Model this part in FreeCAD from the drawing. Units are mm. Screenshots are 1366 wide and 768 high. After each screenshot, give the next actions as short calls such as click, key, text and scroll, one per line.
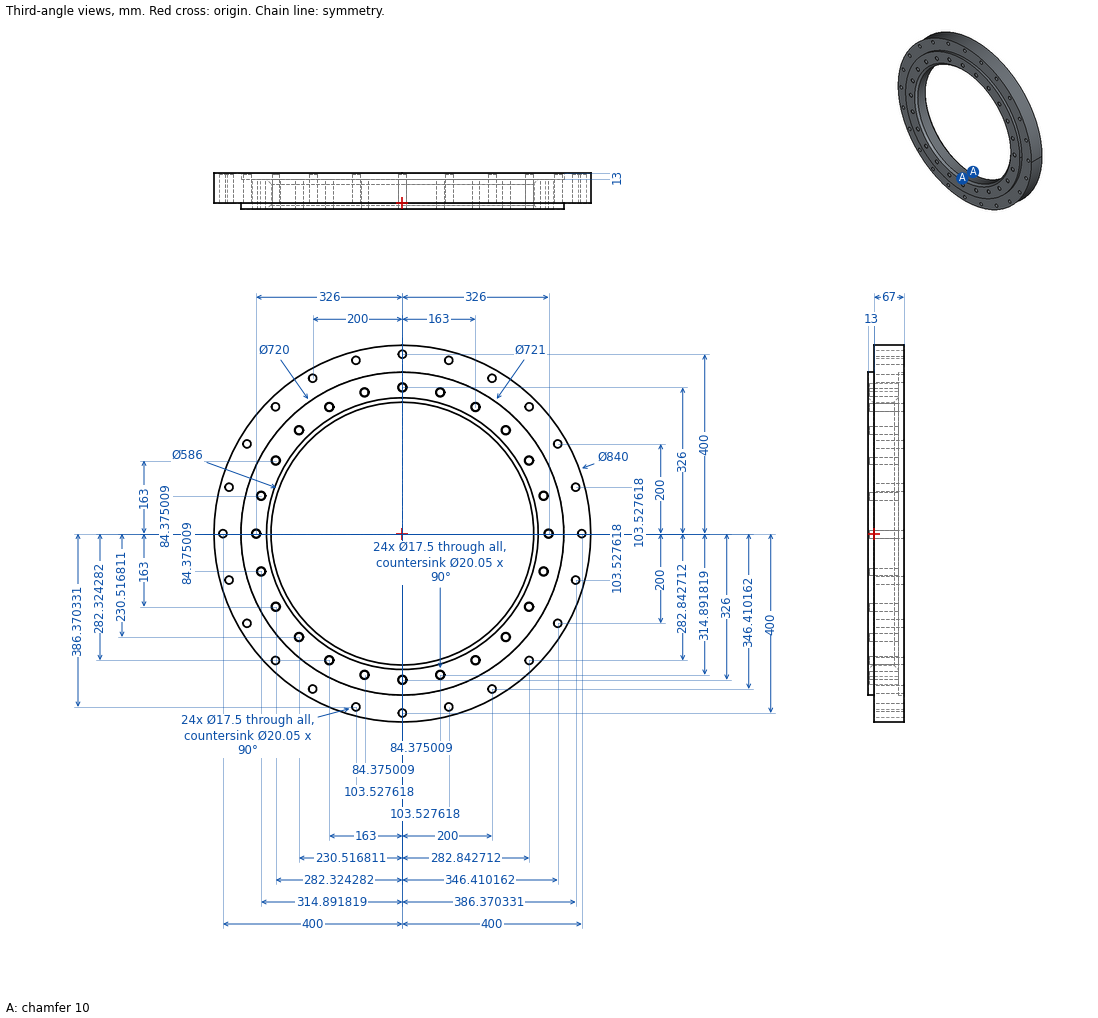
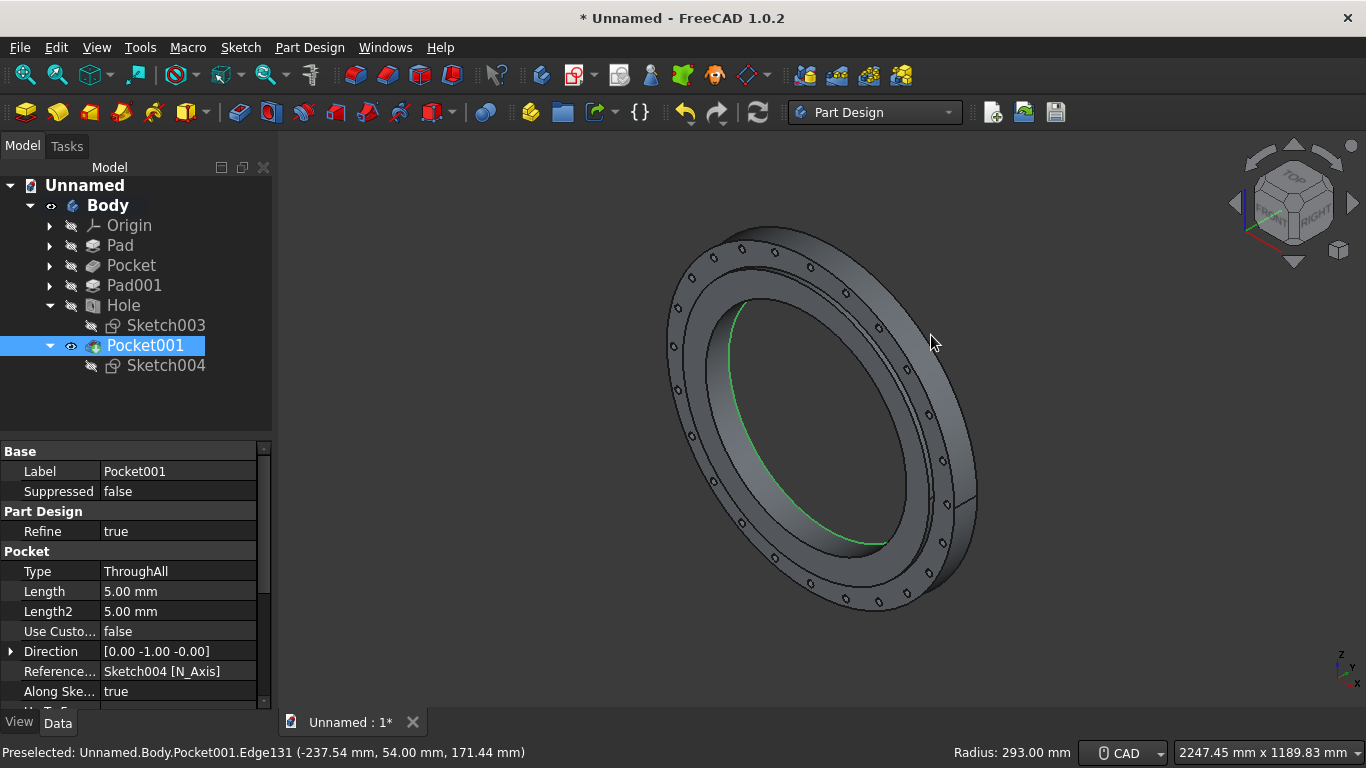
click(706, 369, ctrl)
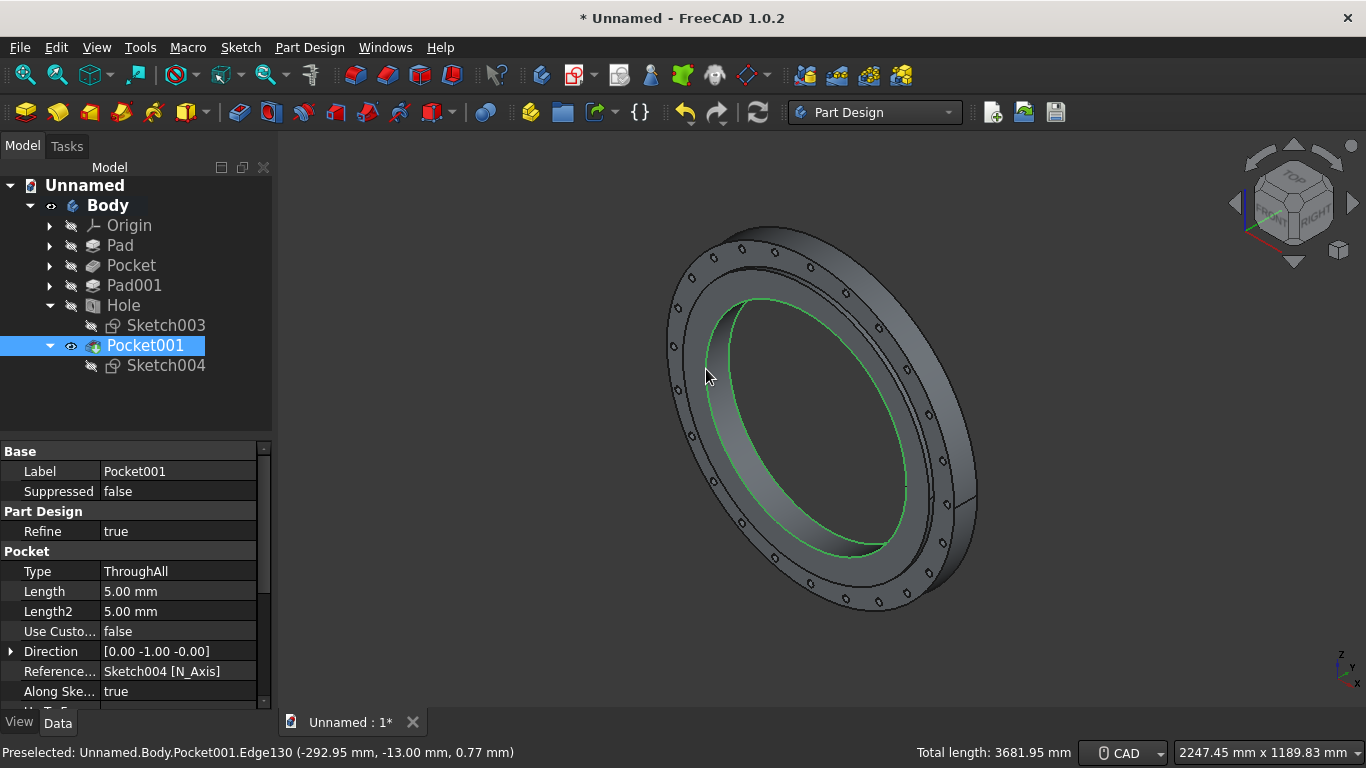
click(388, 76)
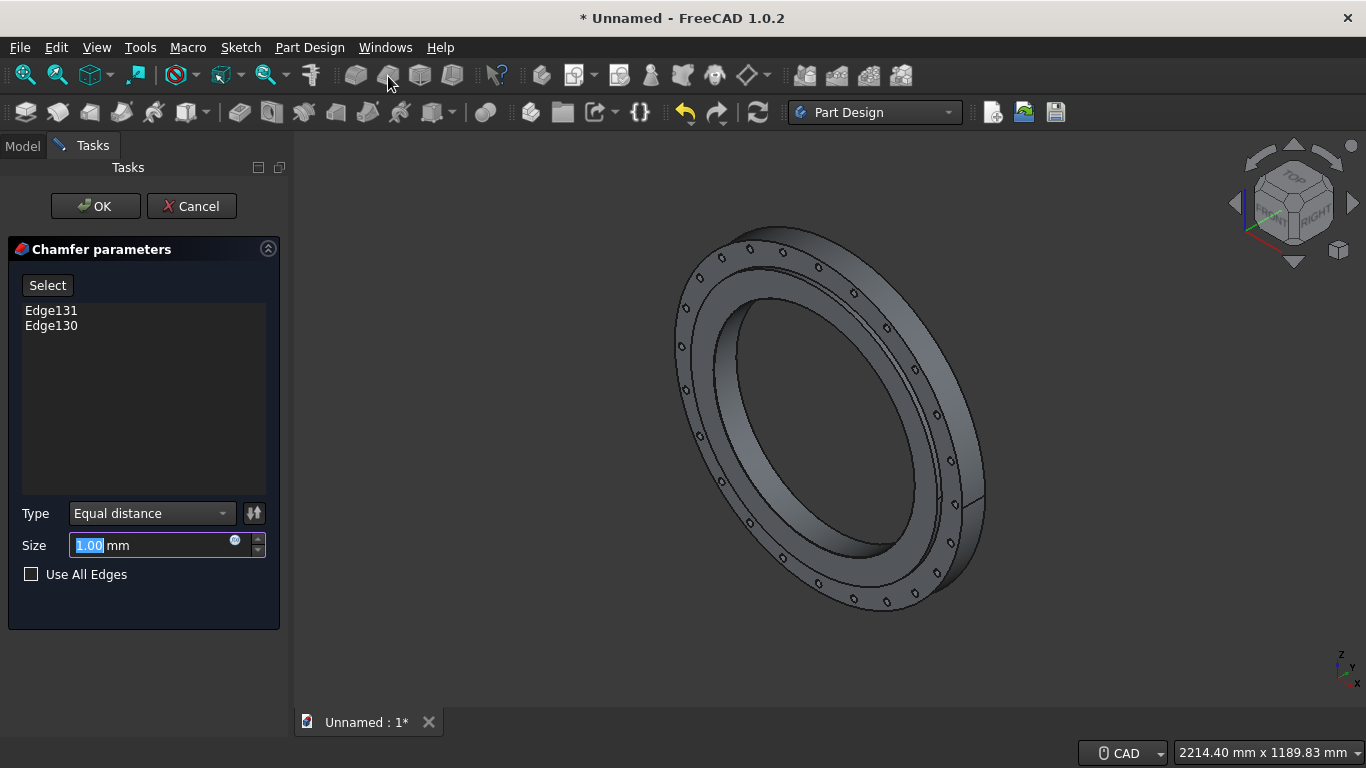
text(10)
key(Tab)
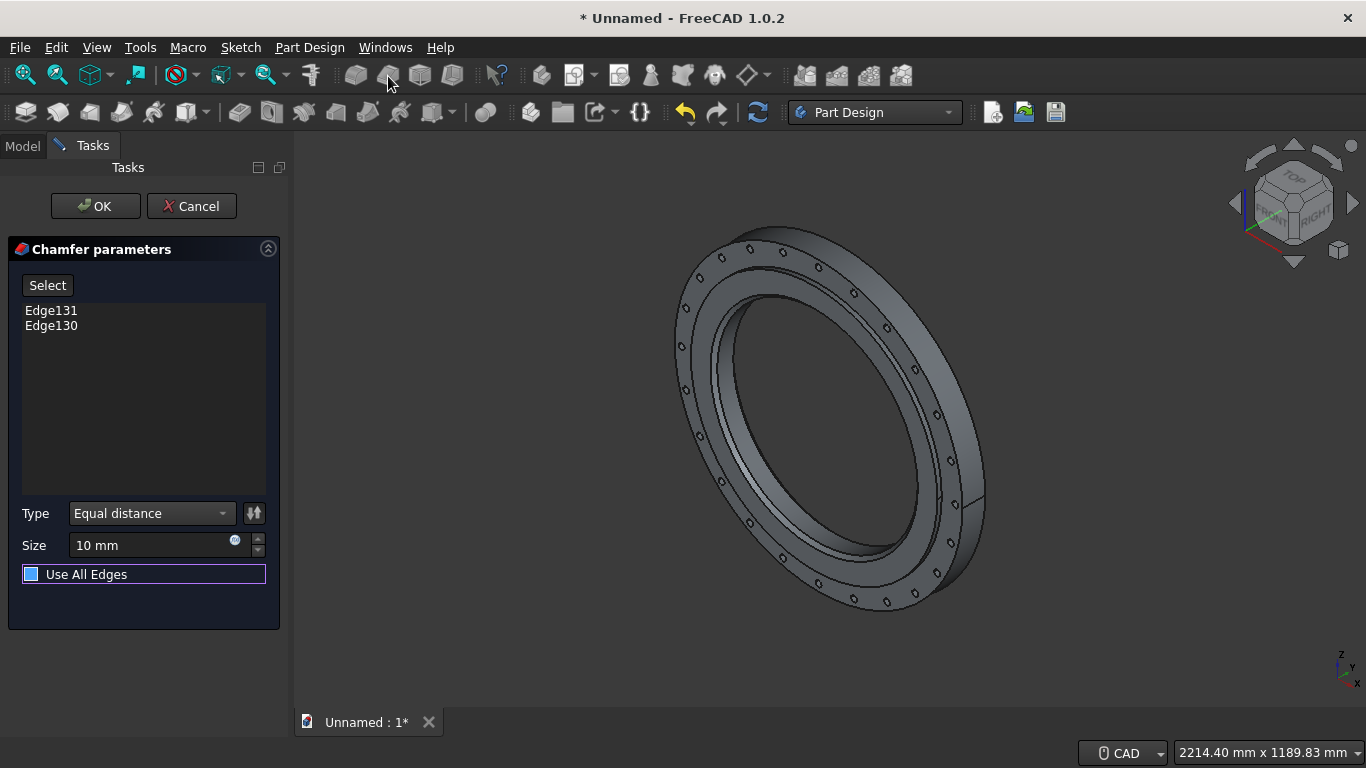
click(96, 206)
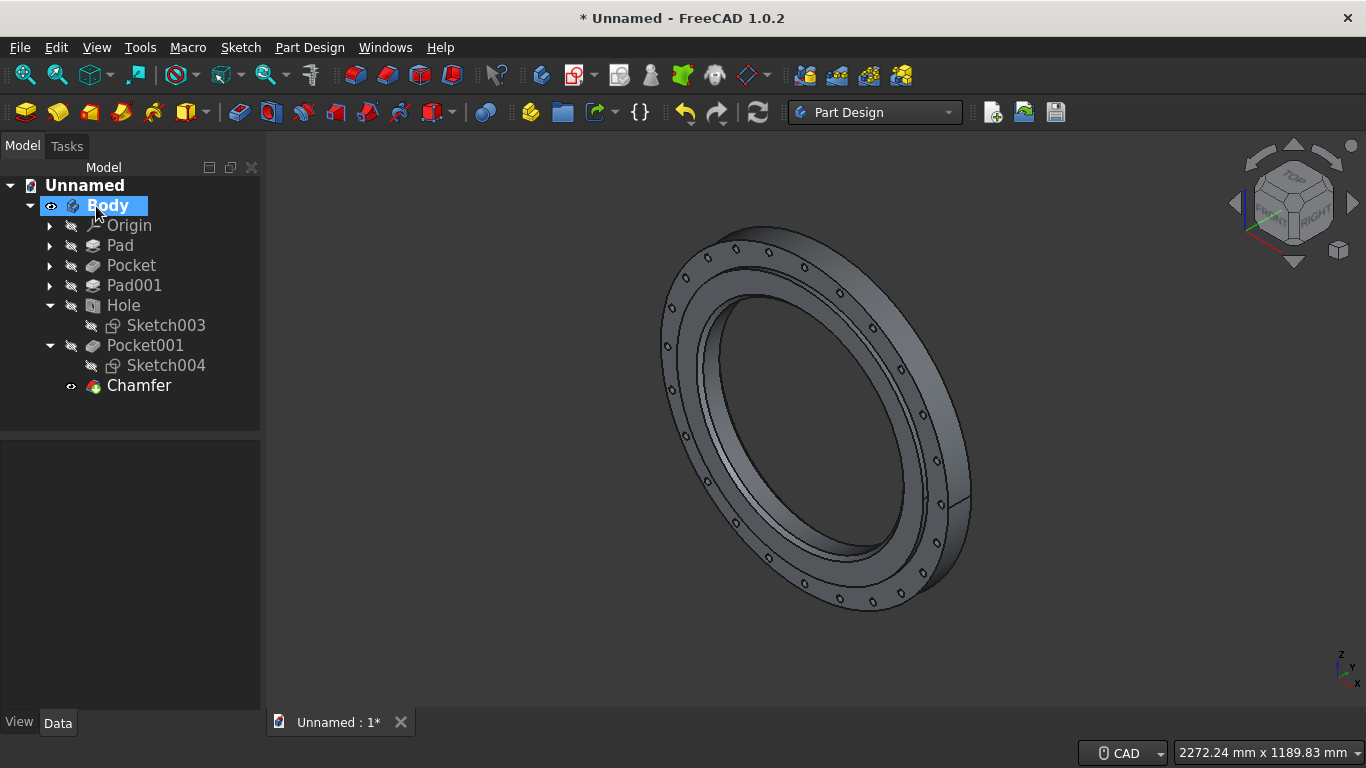
click(835, 569)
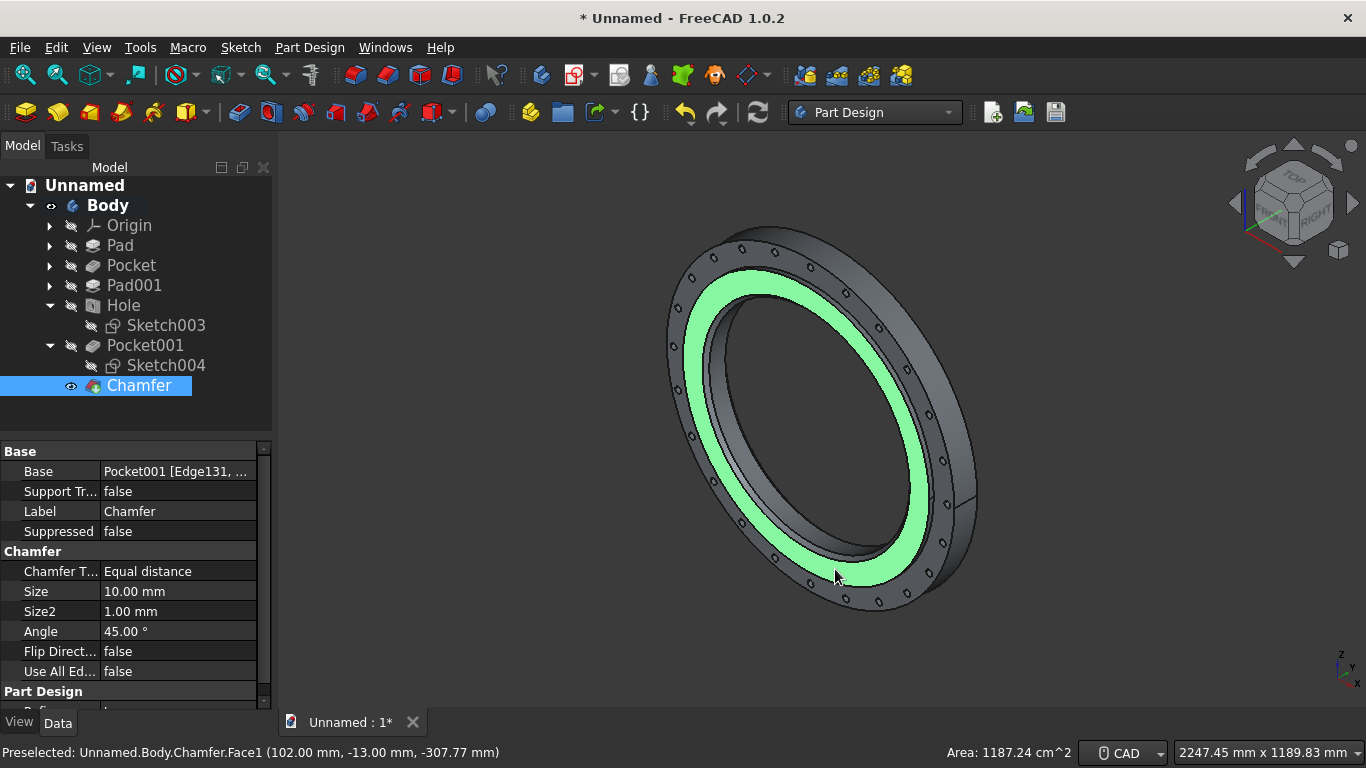
click(574, 76)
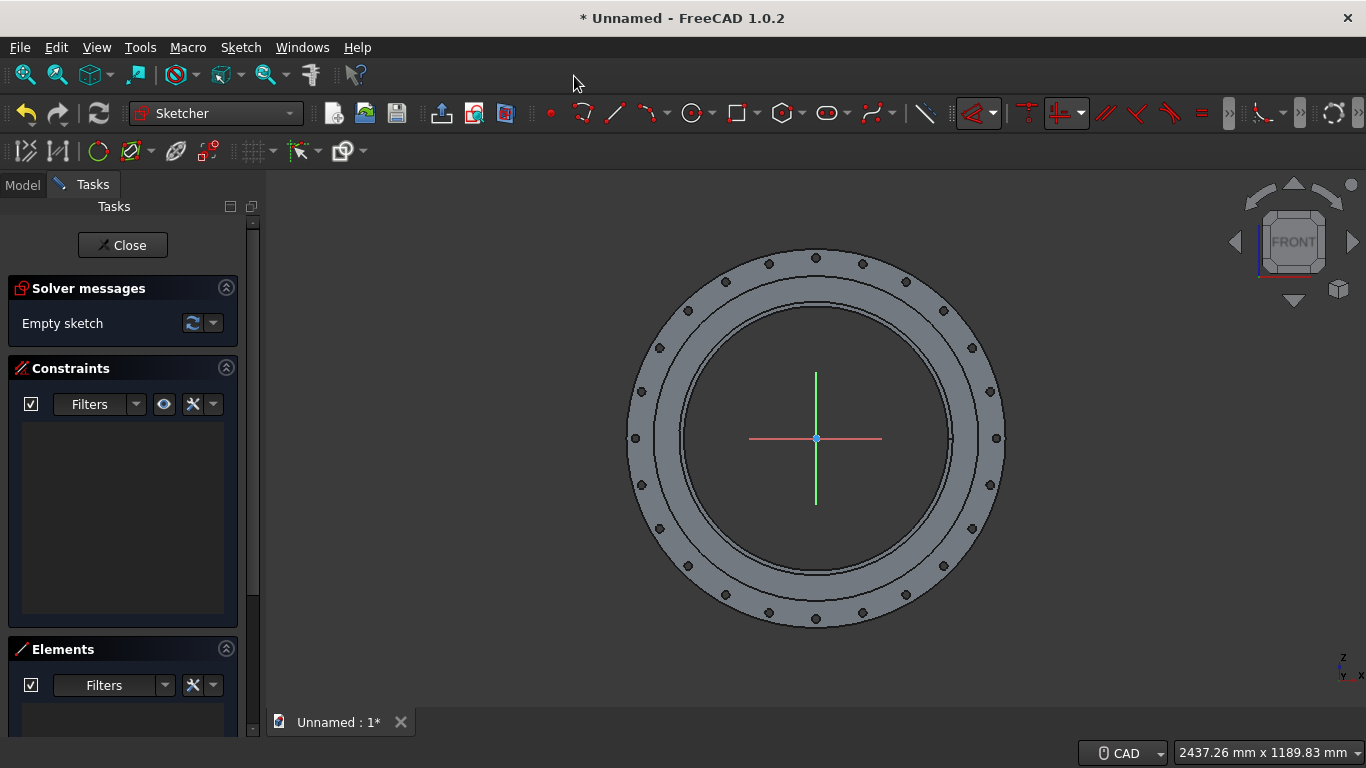
key(g)
key(c)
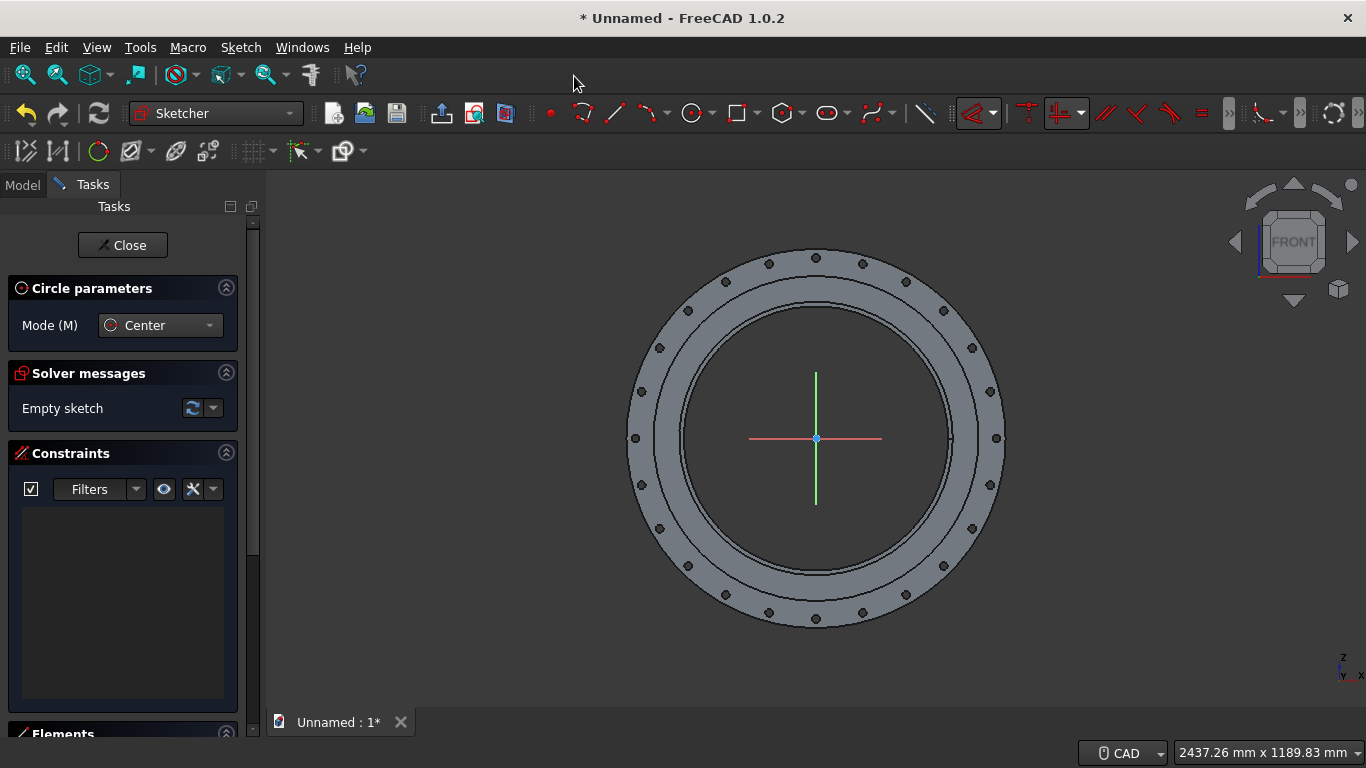
scroll(854, 581, up, 9)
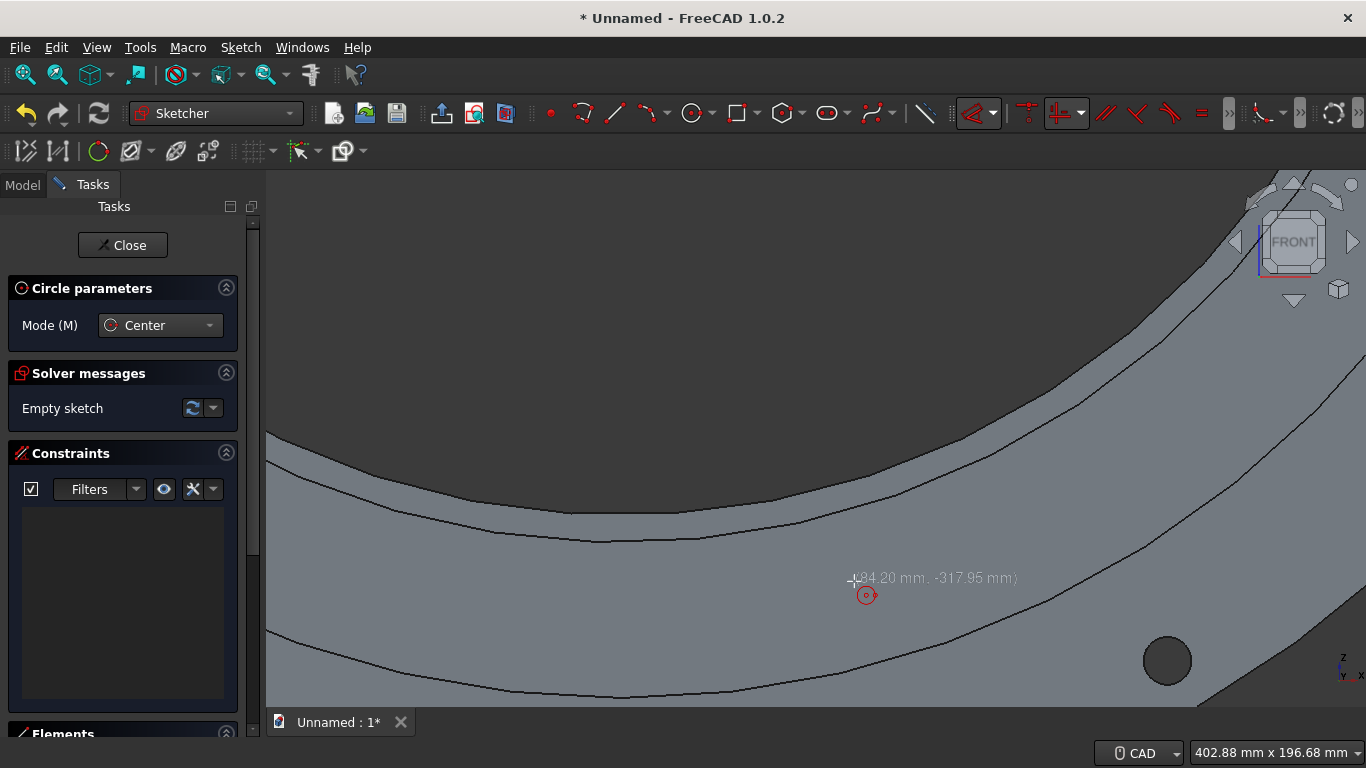
scroll(779, 622, down, 8)